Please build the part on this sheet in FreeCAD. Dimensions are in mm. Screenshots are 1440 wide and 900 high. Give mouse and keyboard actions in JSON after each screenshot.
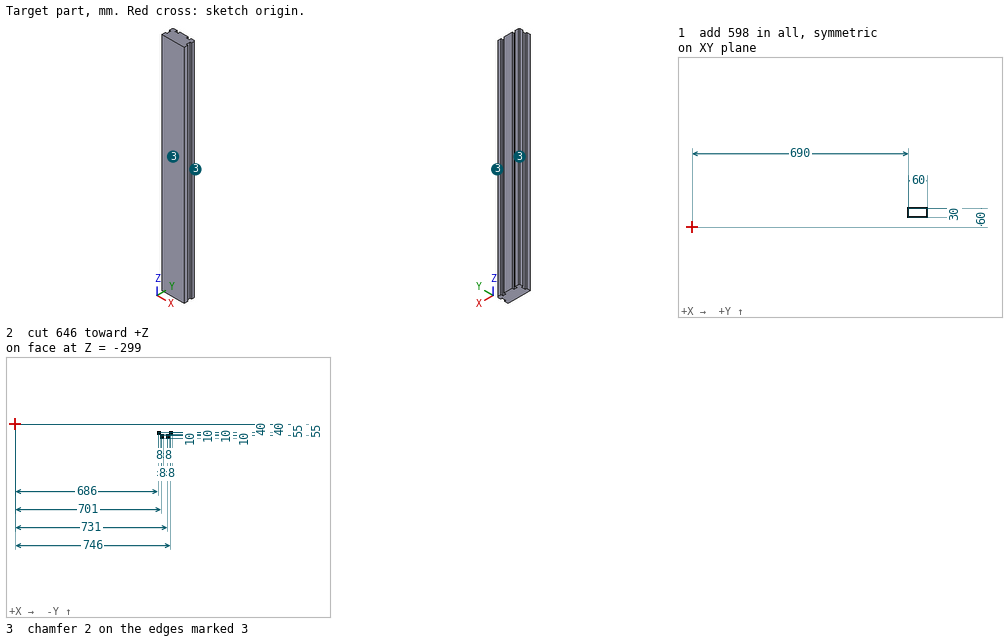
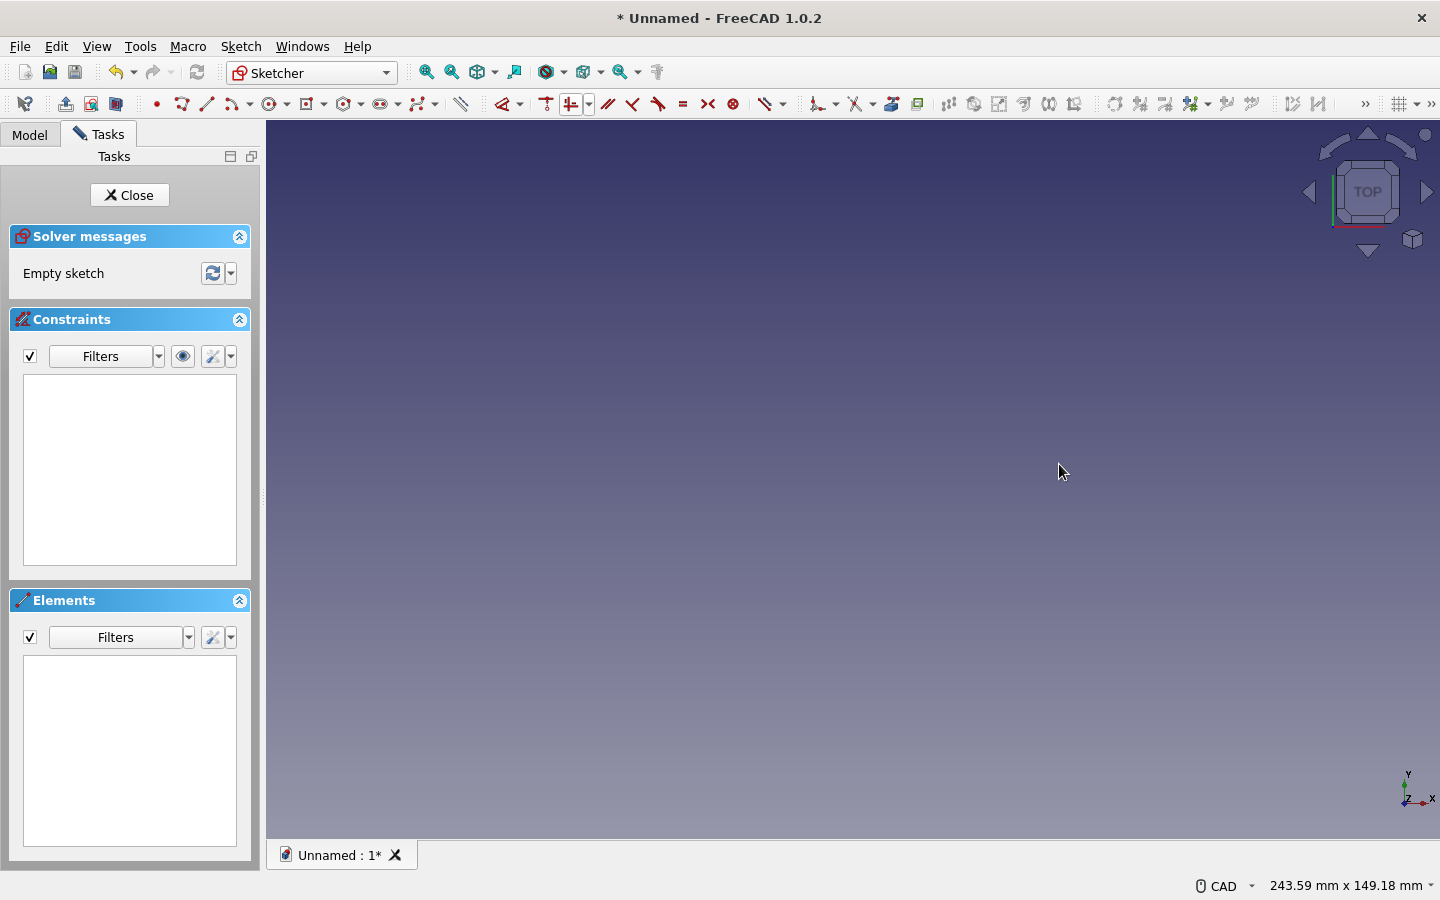
{"action": "scroll", "coordinate": [761, 426], "scroll_direction": "up", "scroll_amount": 2}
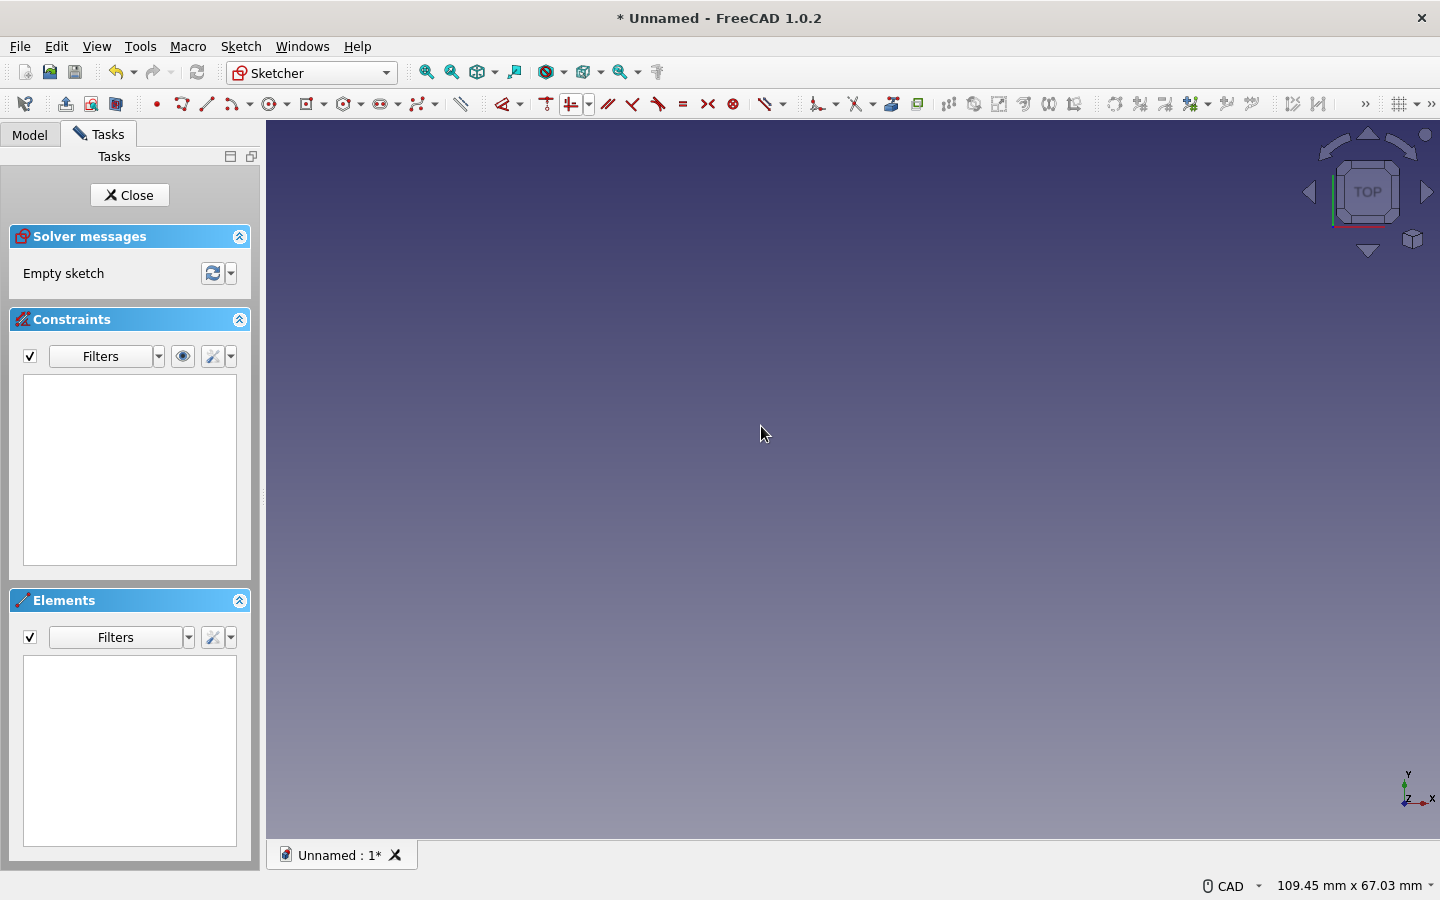
{"action": "key", "text": "g r"}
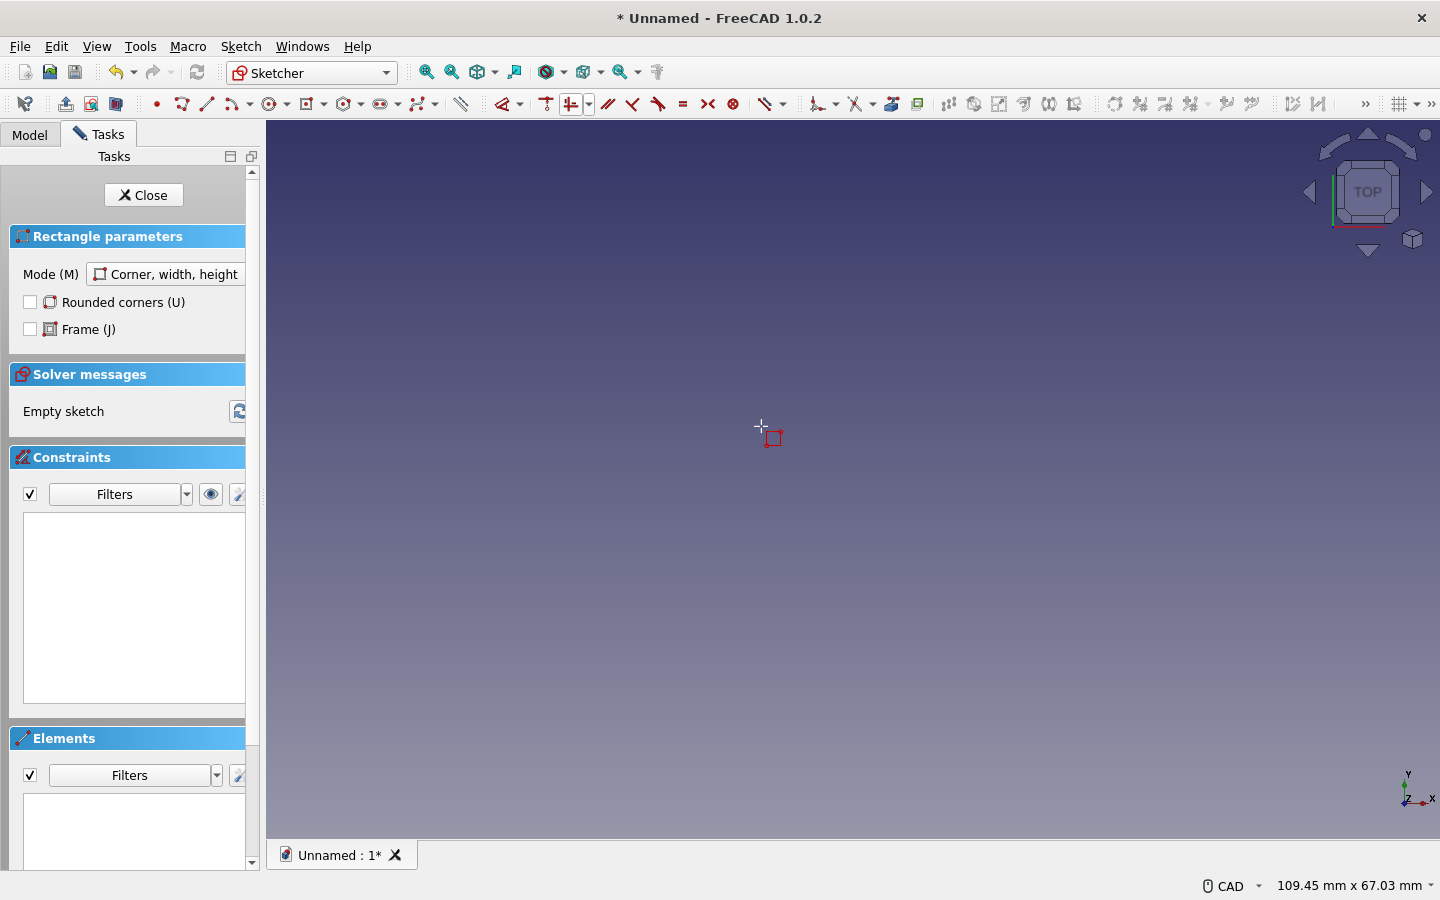
{"action": "left_click", "coordinate": [463, 318]}
{"action": "left_click", "coordinate": [1106, 640]}
{"action": "key", "text": "Escape"}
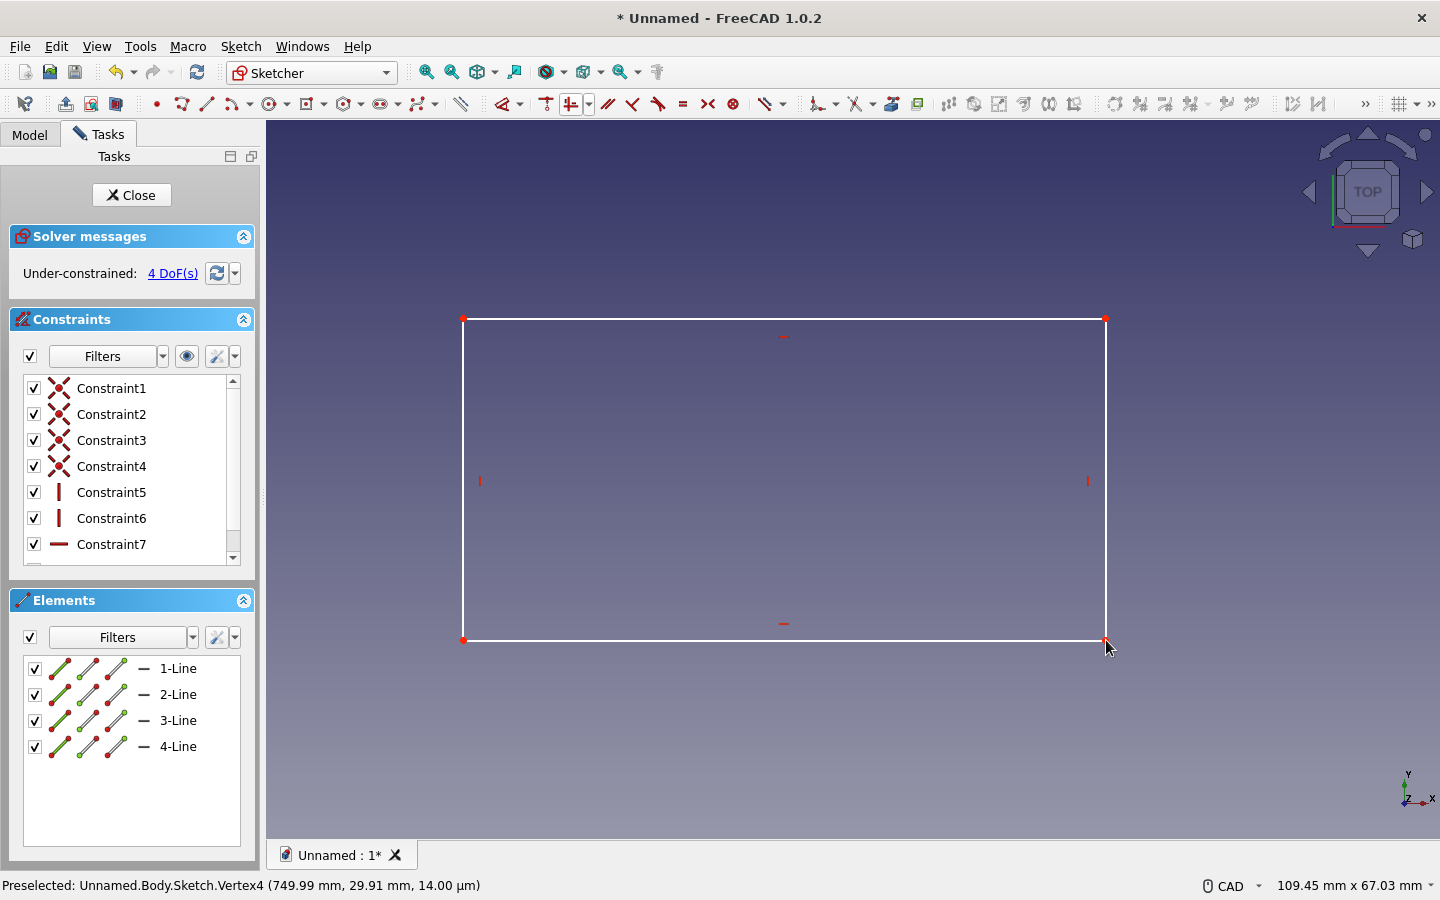
{"action": "left_click", "coordinate": [502, 104]}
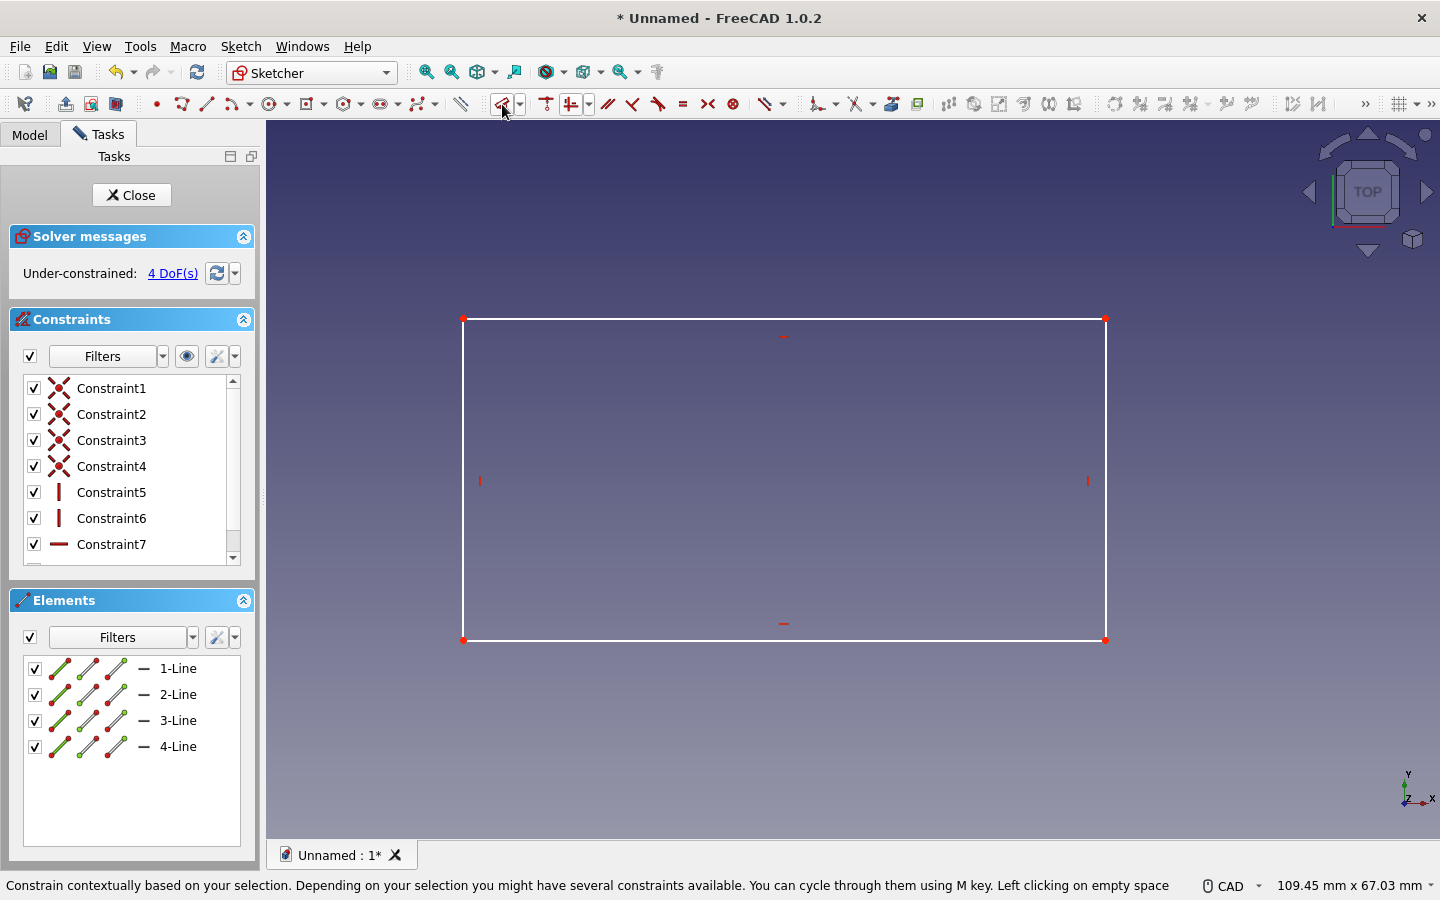
{"action": "left_click", "coordinate": [463, 416]}
{"action": "left_click", "coordinate": [429, 480]}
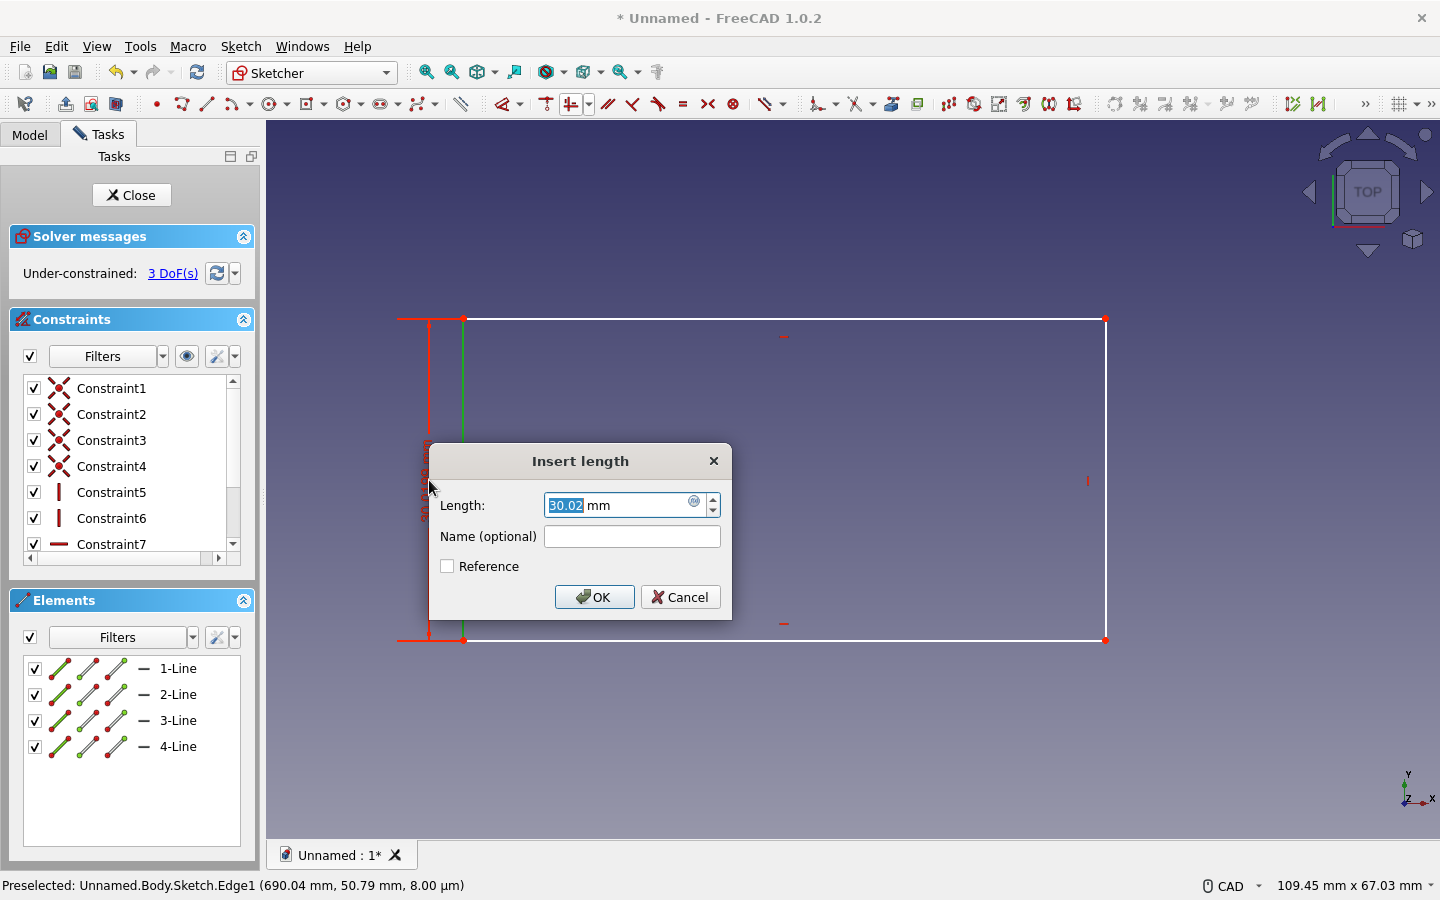
{"action": "type", "text": "30"}
{"action": "key", "text": "Return"}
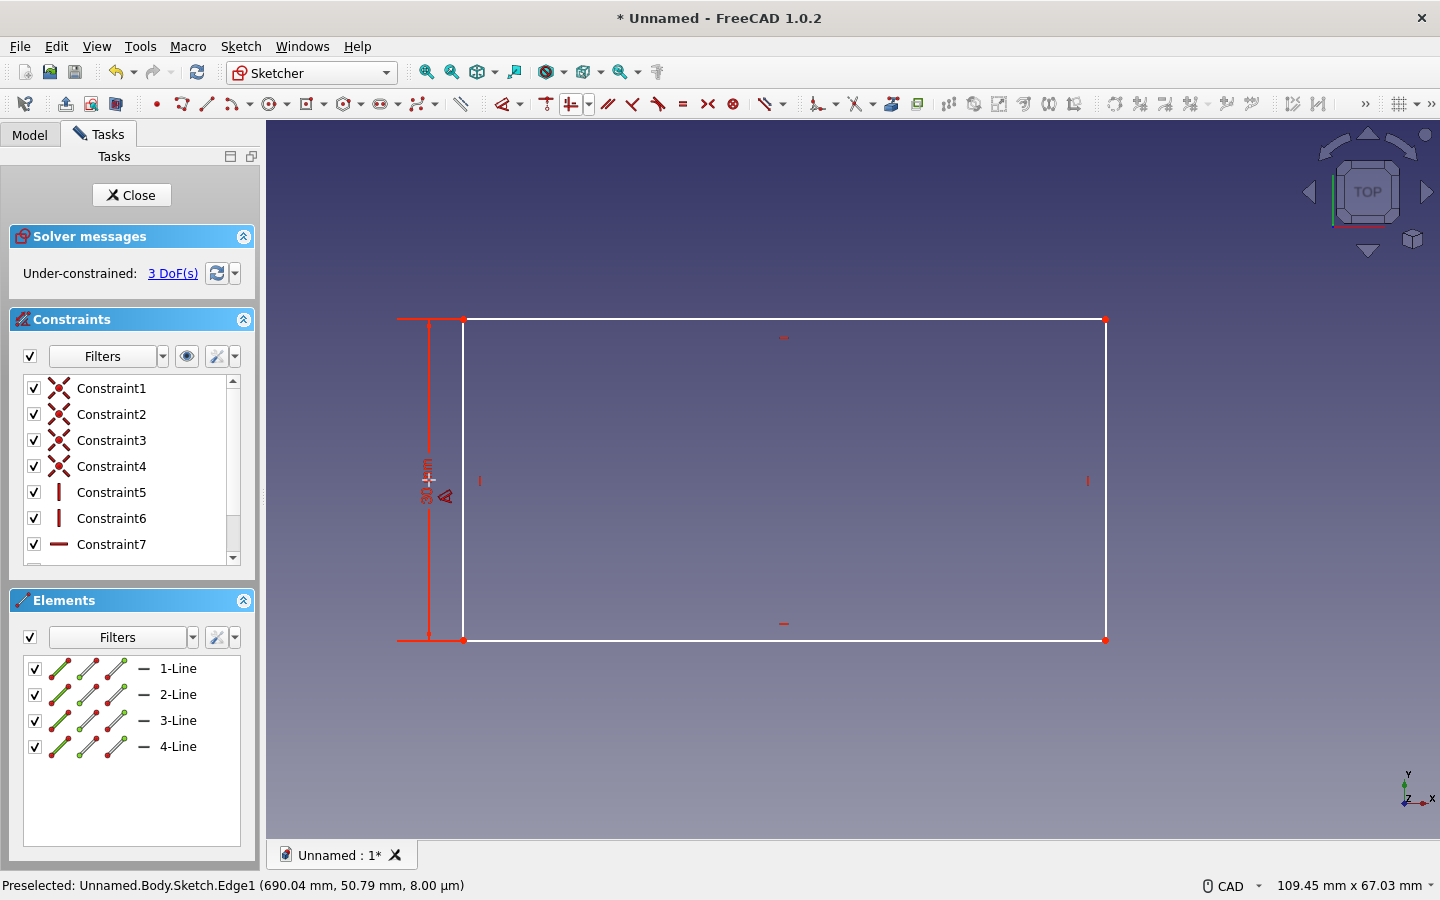
{"action": "left_click", "coordinate": [656, 641]}
{"action": "left_click", "coordinate": [784, 675]}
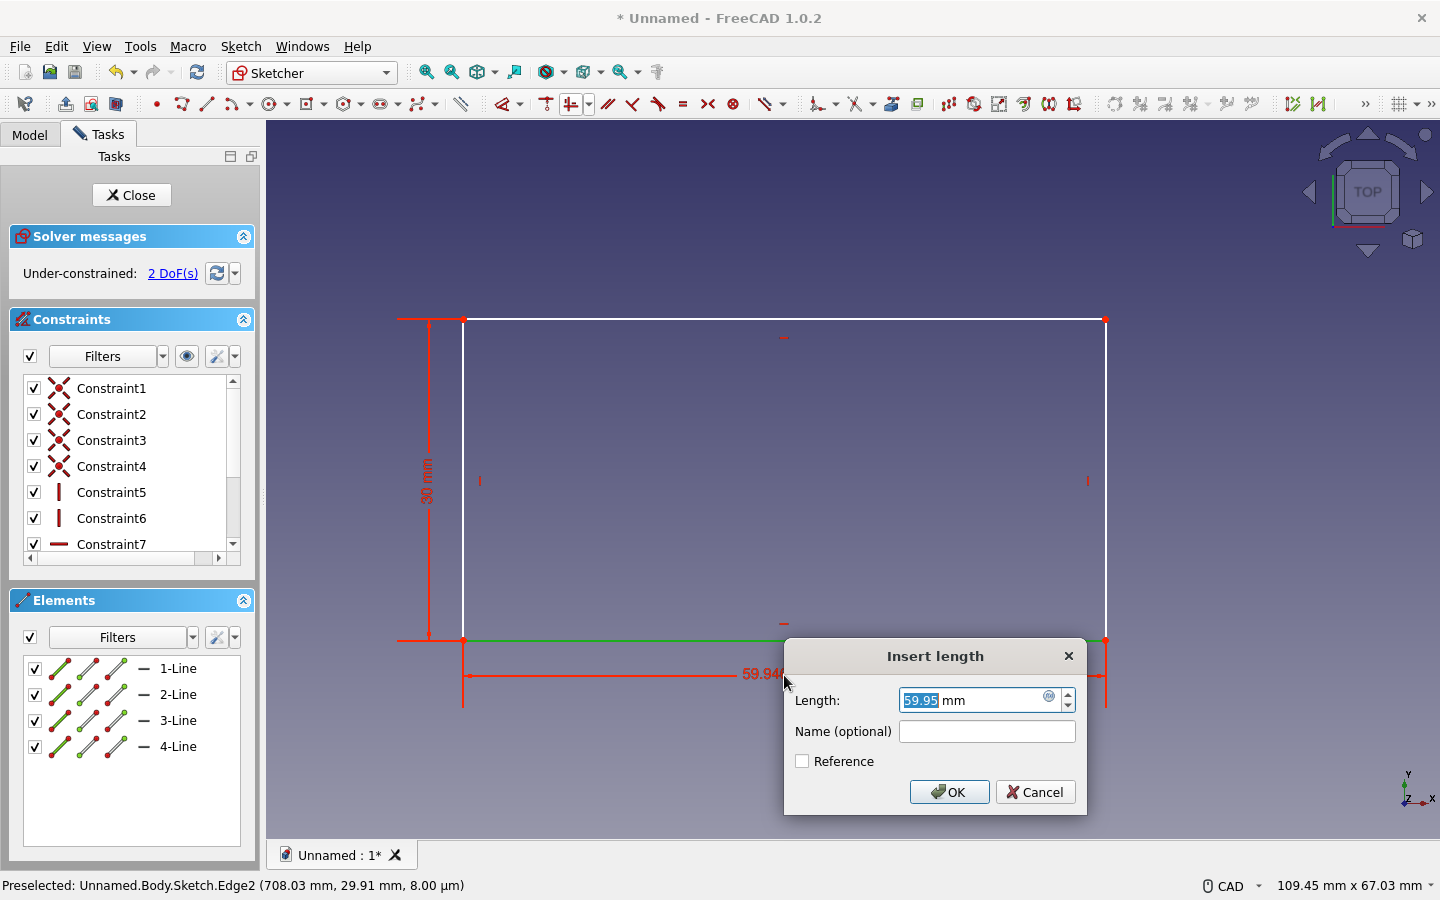
{"action": "type", "text": "60"}
{"action": "key", "text": "Return"}